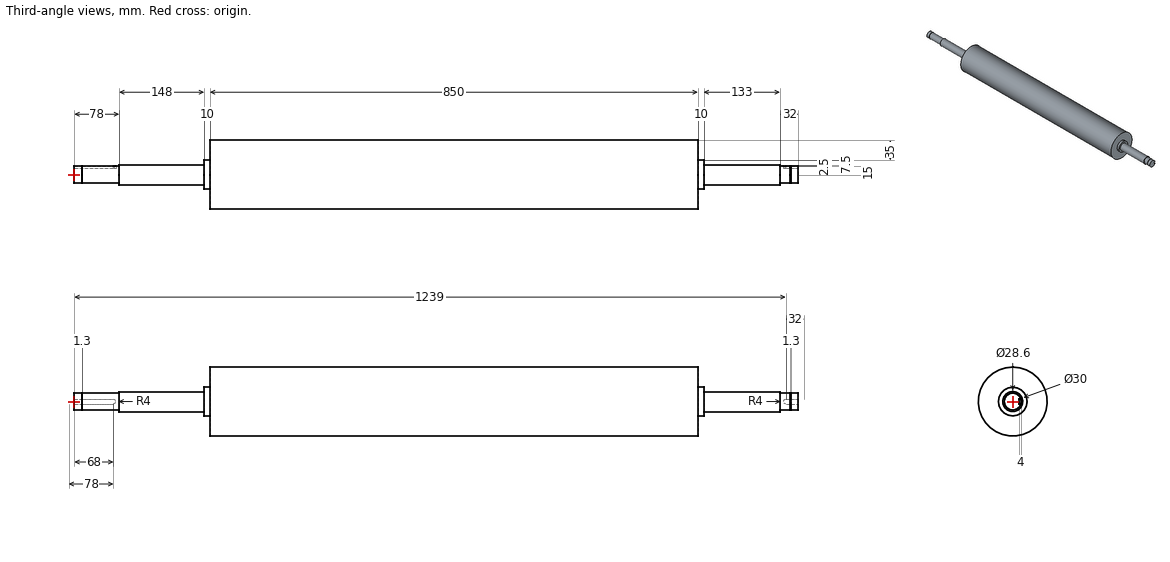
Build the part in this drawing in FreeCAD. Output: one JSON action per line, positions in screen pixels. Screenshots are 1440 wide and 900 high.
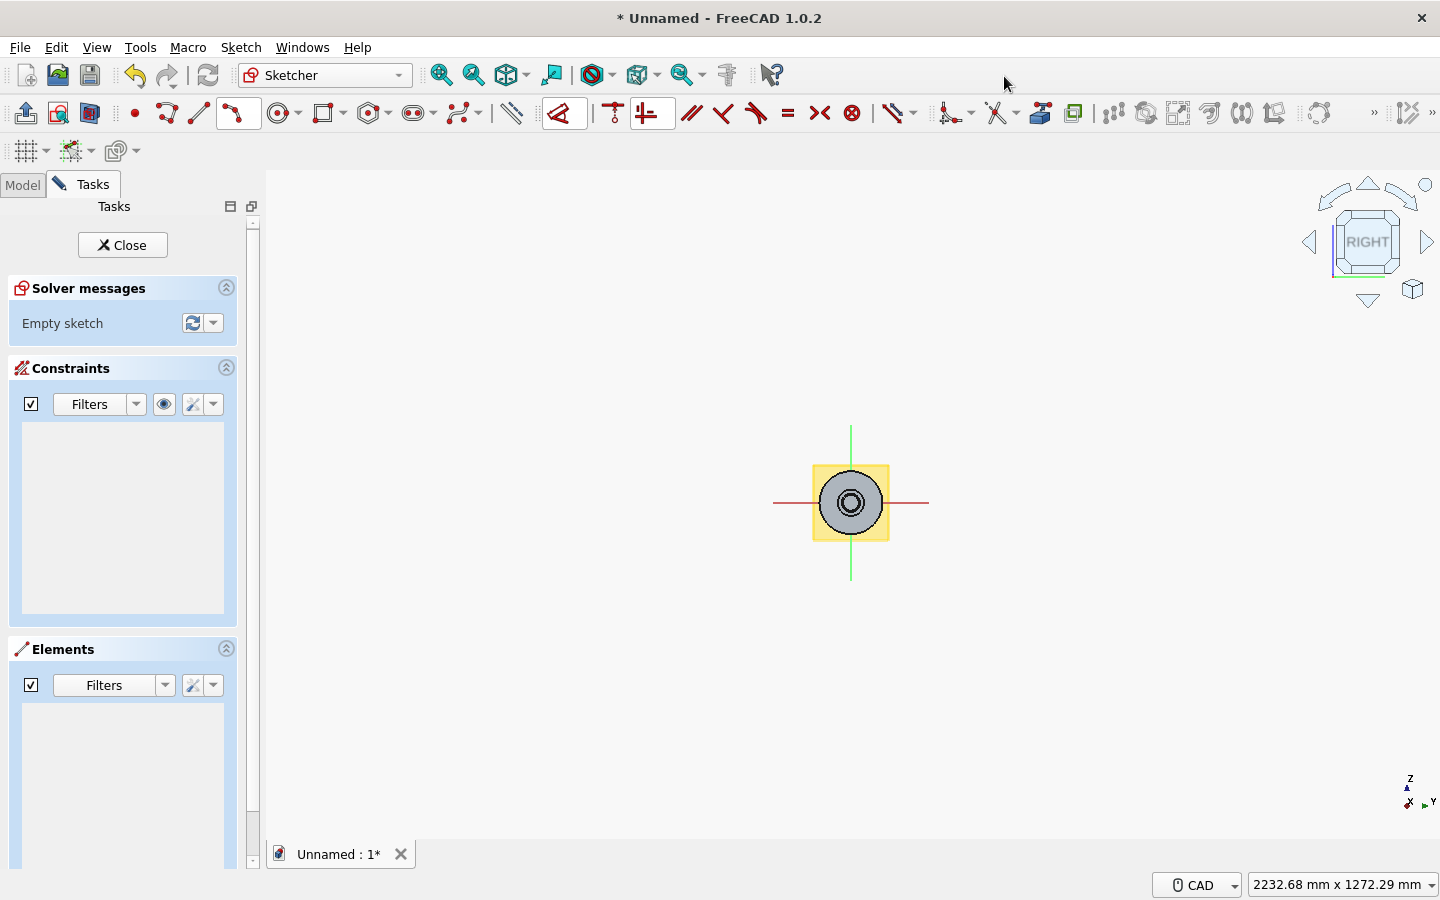
{"action": "left_click", "coordinate": [90, 114]}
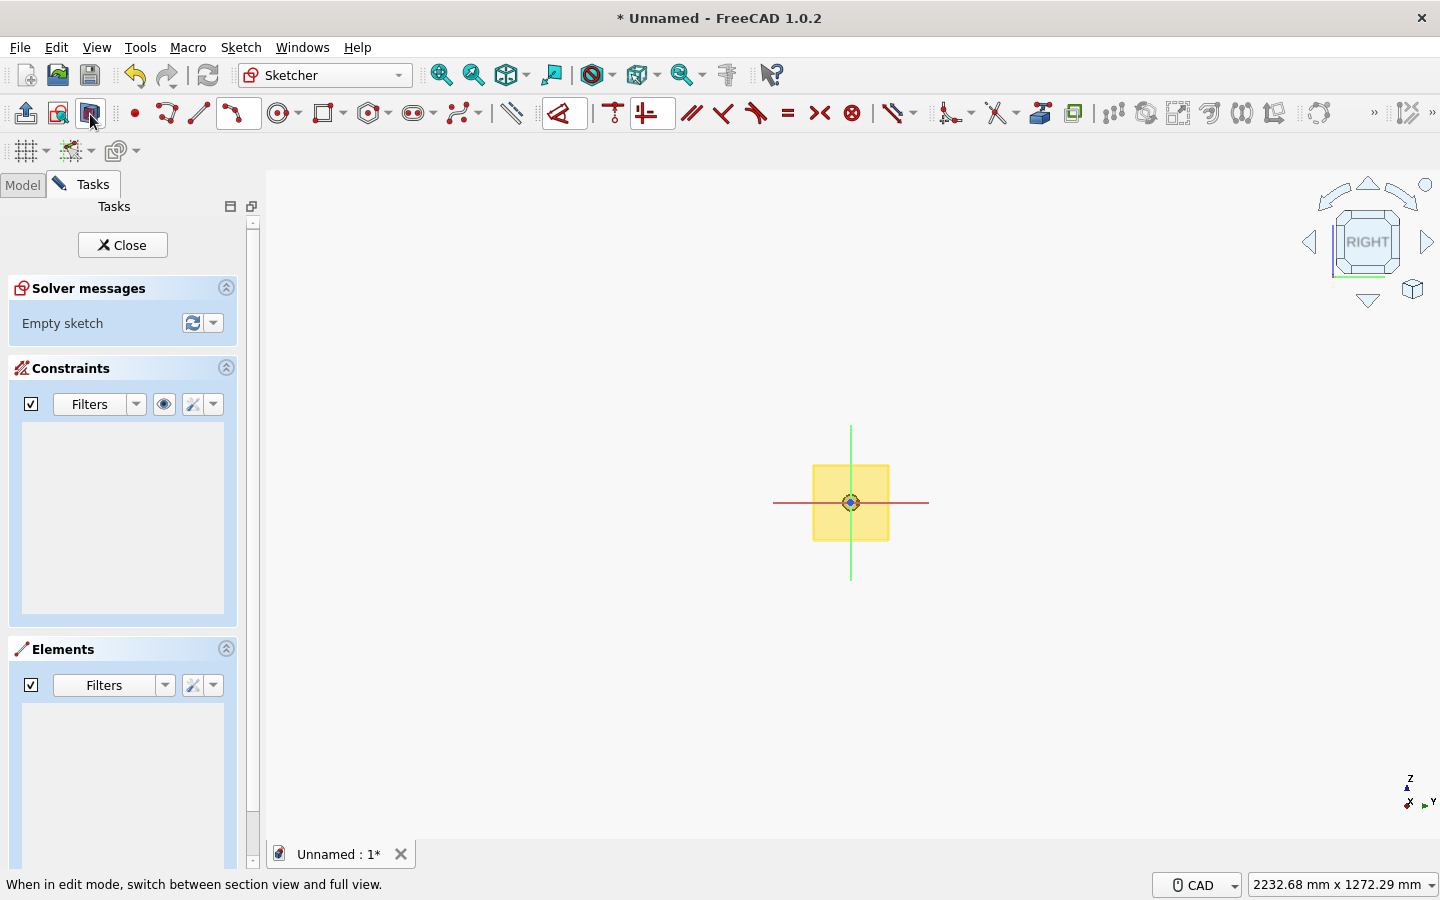
{"action": "scroll", "coordinate": [854, 503], "scroll_direction": "up", "scroll_amount": 15}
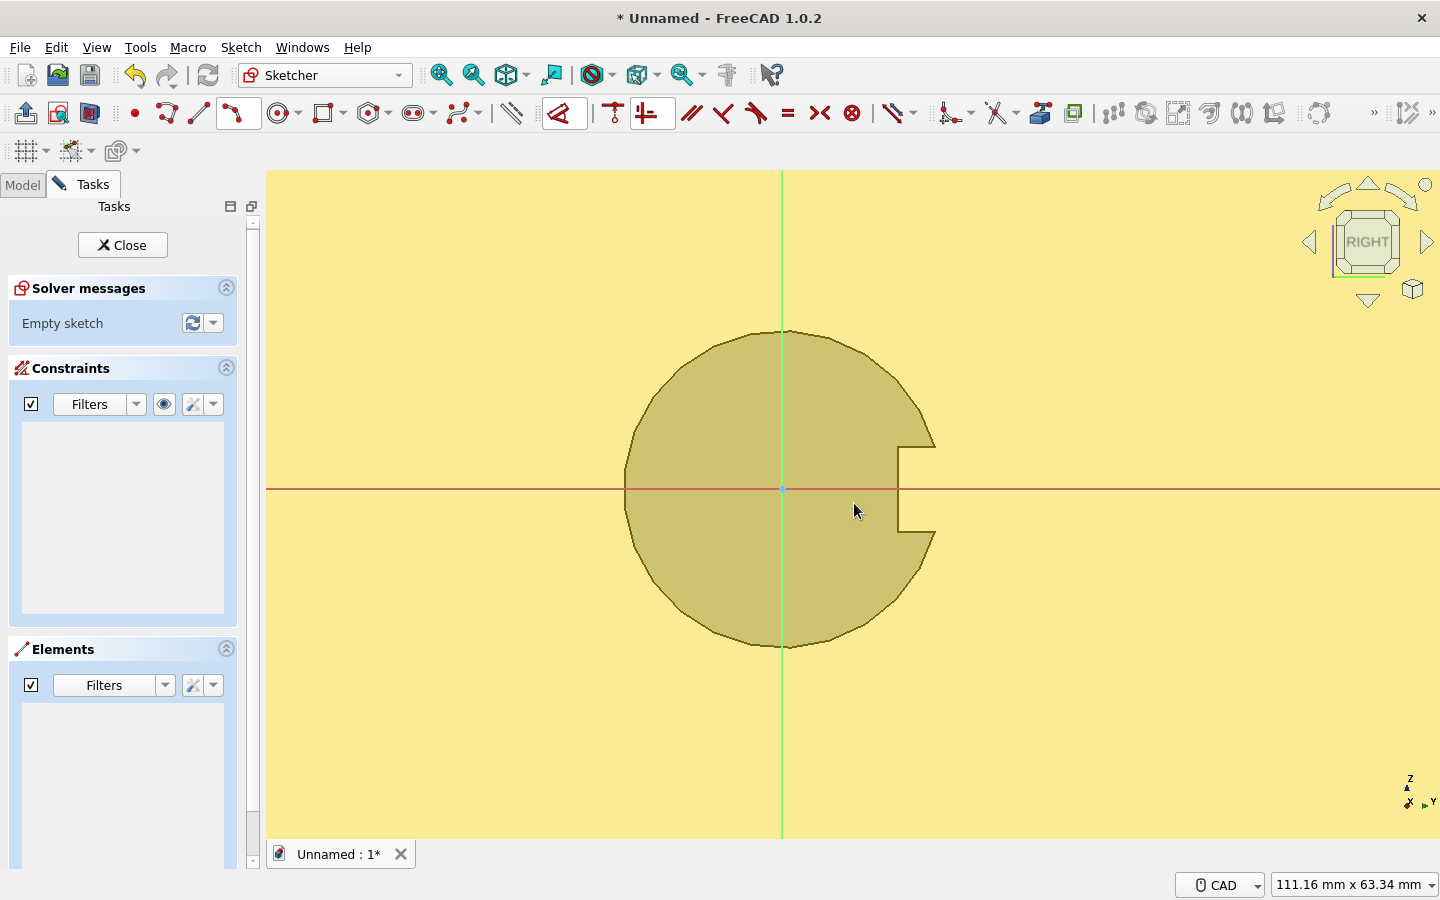
{"action": "scroll", "coordinate": [777, 459], "scroll_direction": "up", "scroll_amount": 2}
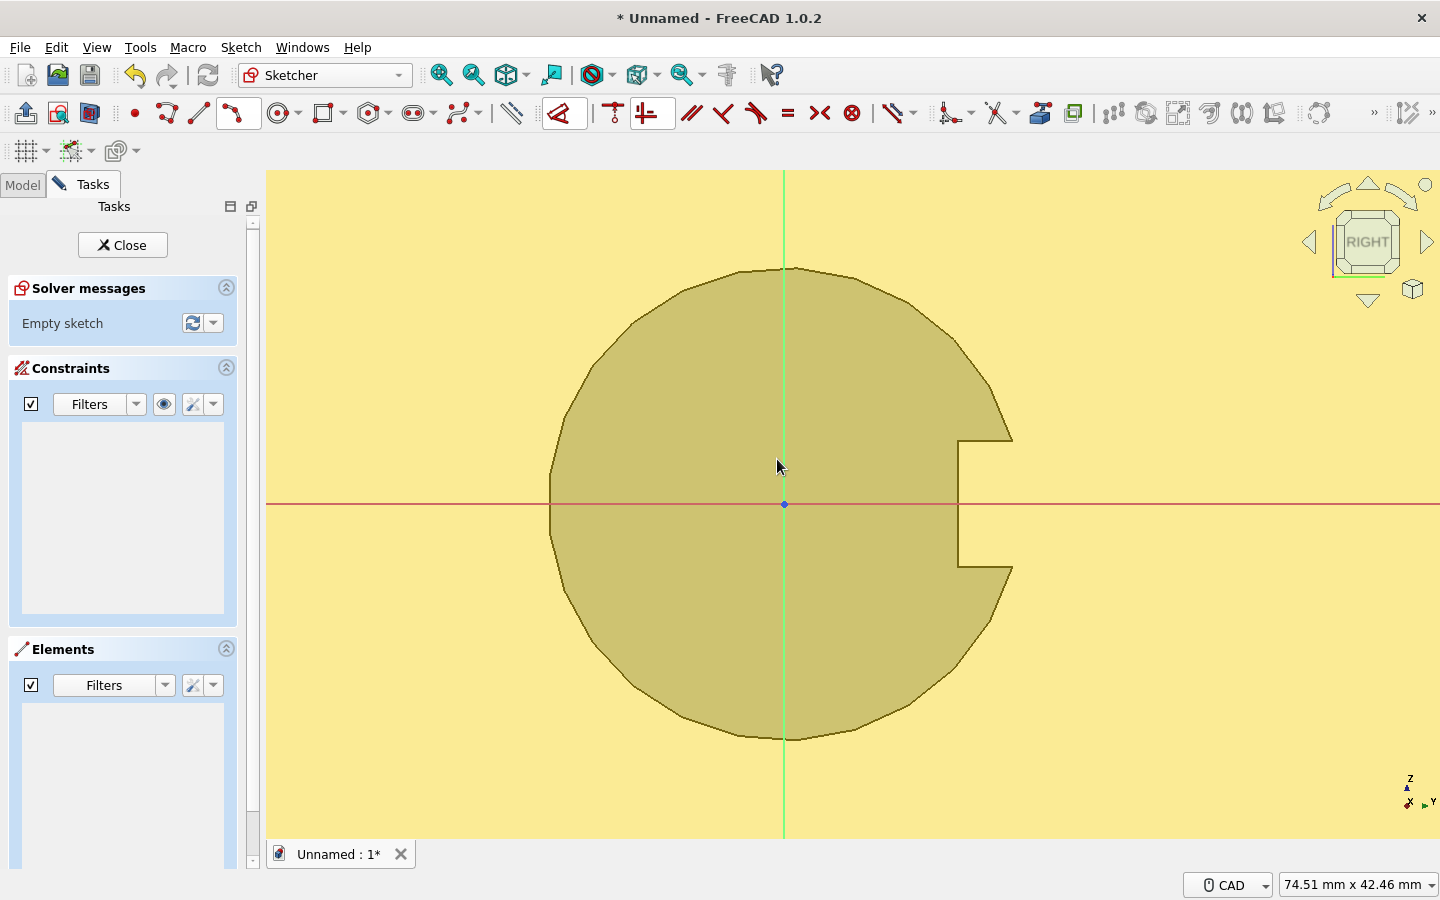
{"action": "left_click", "coordinate": [278, 114]}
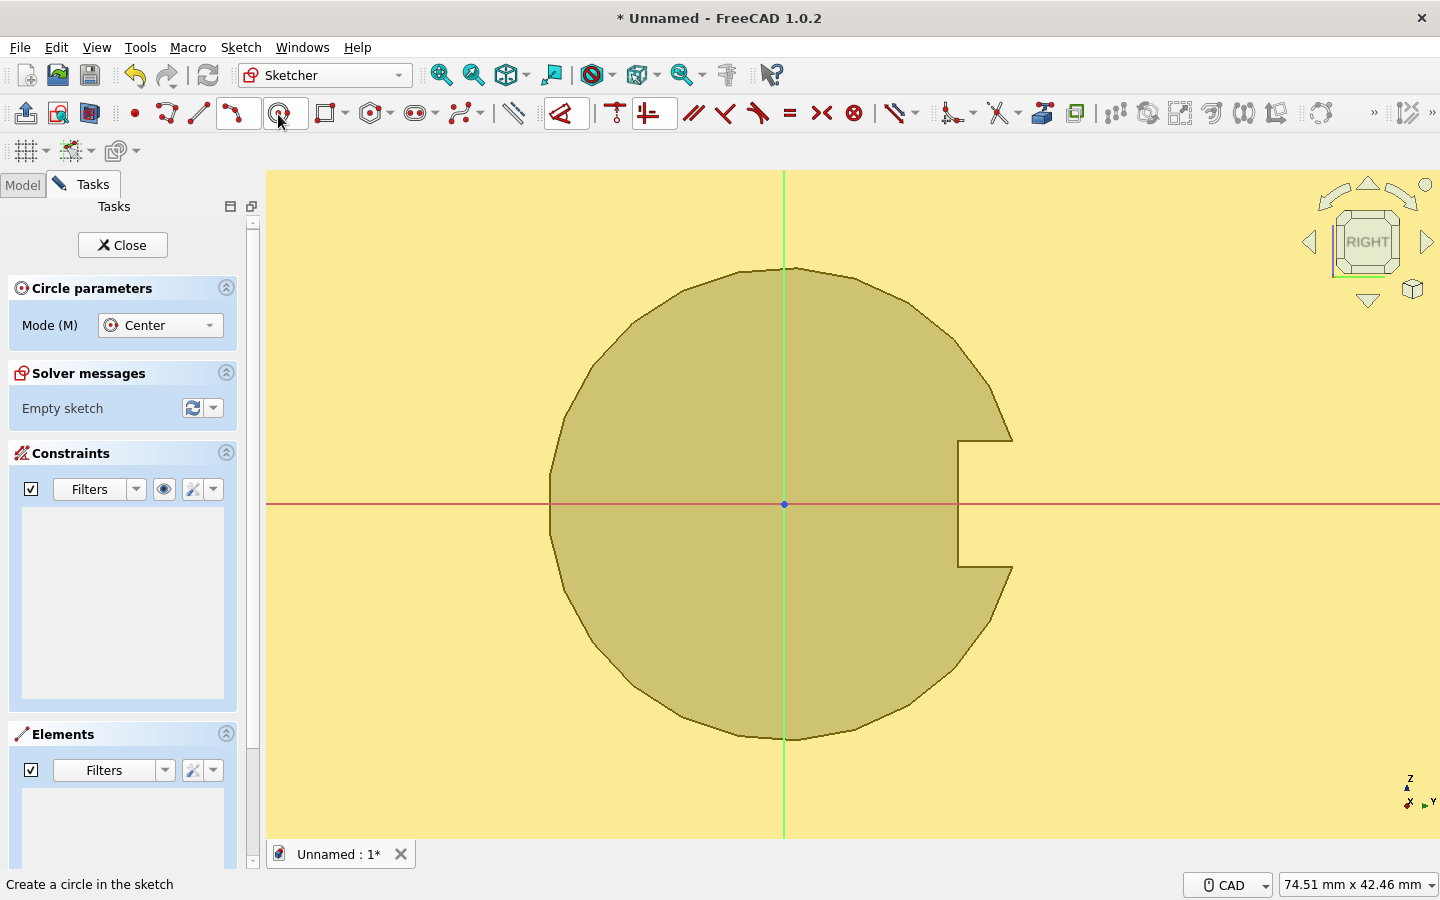
{"action": "left_click", "coordinate": [784, 504]}
{"action": "mouse_move", "coordinate": [952, 337]}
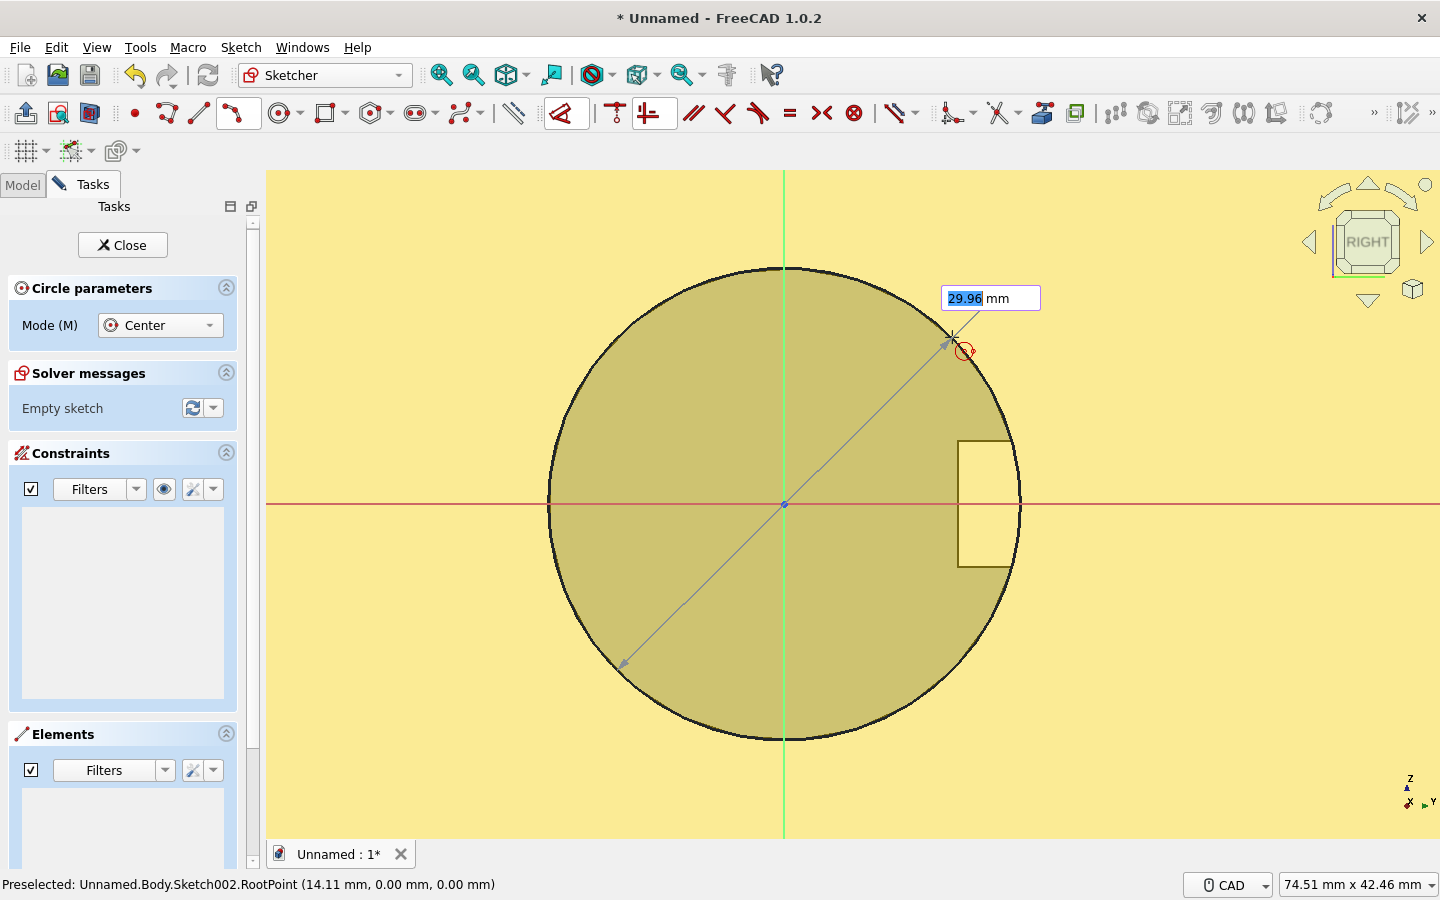
{"action": "type", "text": "30"}
{"action": "key", "text": "Return"}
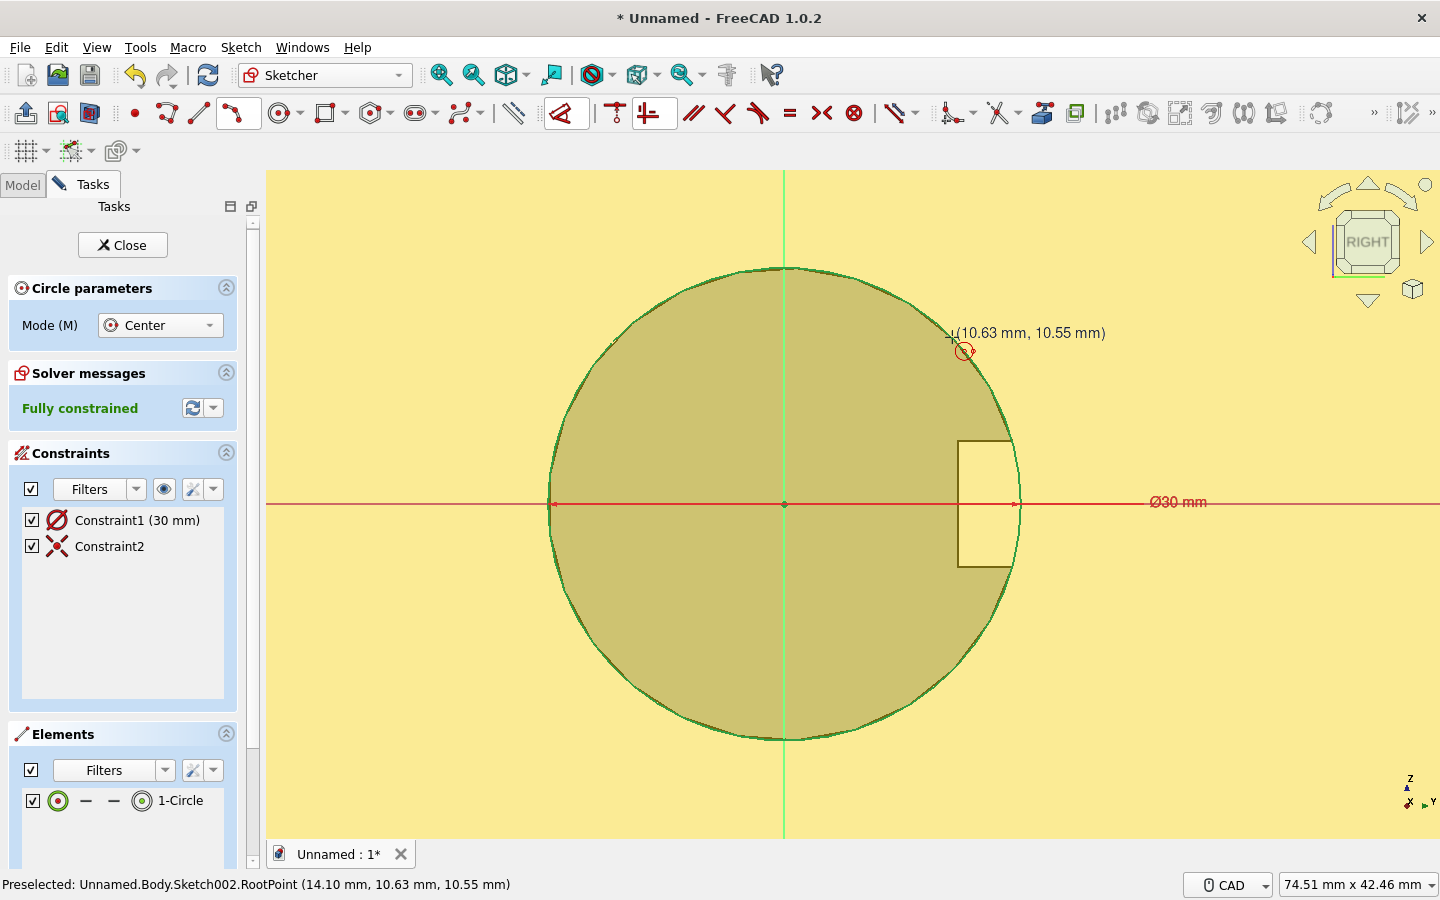
{"action": "left_click", "coordinate": [784, 504]}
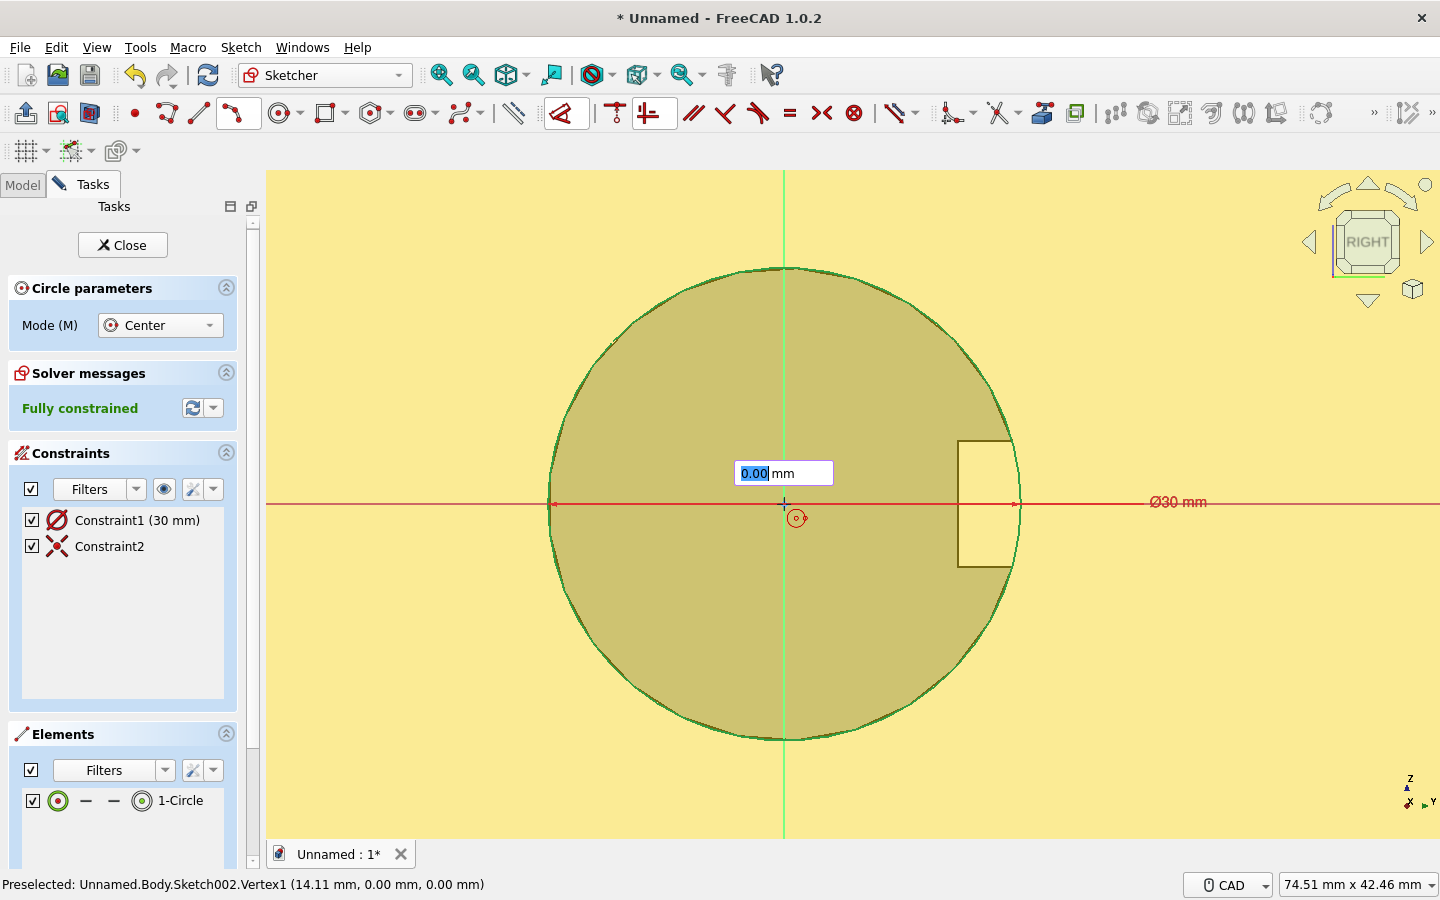
{"action": "scroll", "coordinate": [862, 293], "scroll_direction": "up", "scroll_amount": 2}
{"action": "mouse_move", "coordinate": [861, 292]}